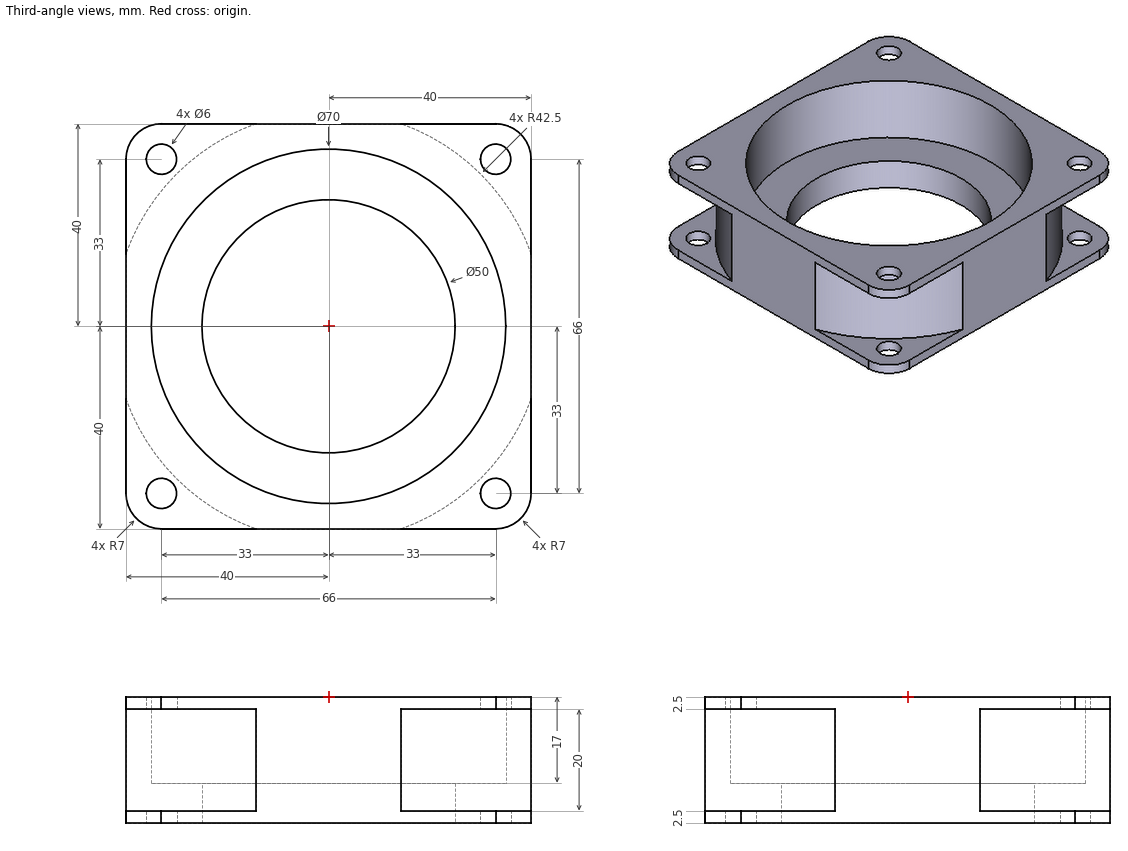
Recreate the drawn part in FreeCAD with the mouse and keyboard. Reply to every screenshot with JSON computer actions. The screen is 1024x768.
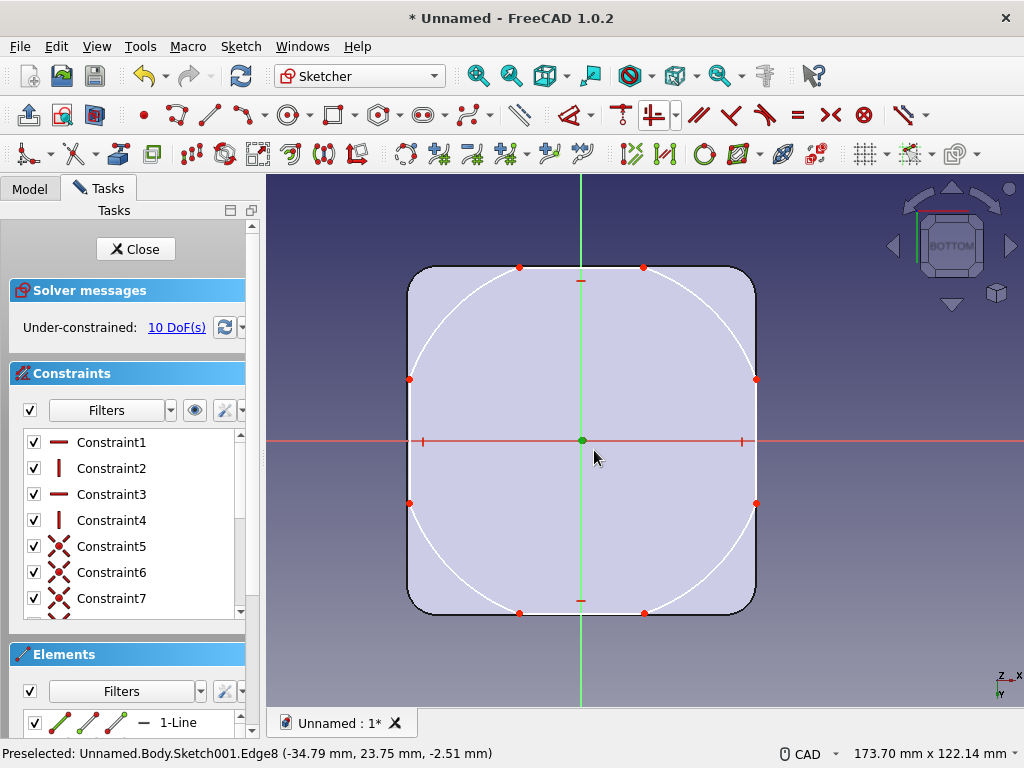
{"action": "left_click", "coordinate": [621, 116]}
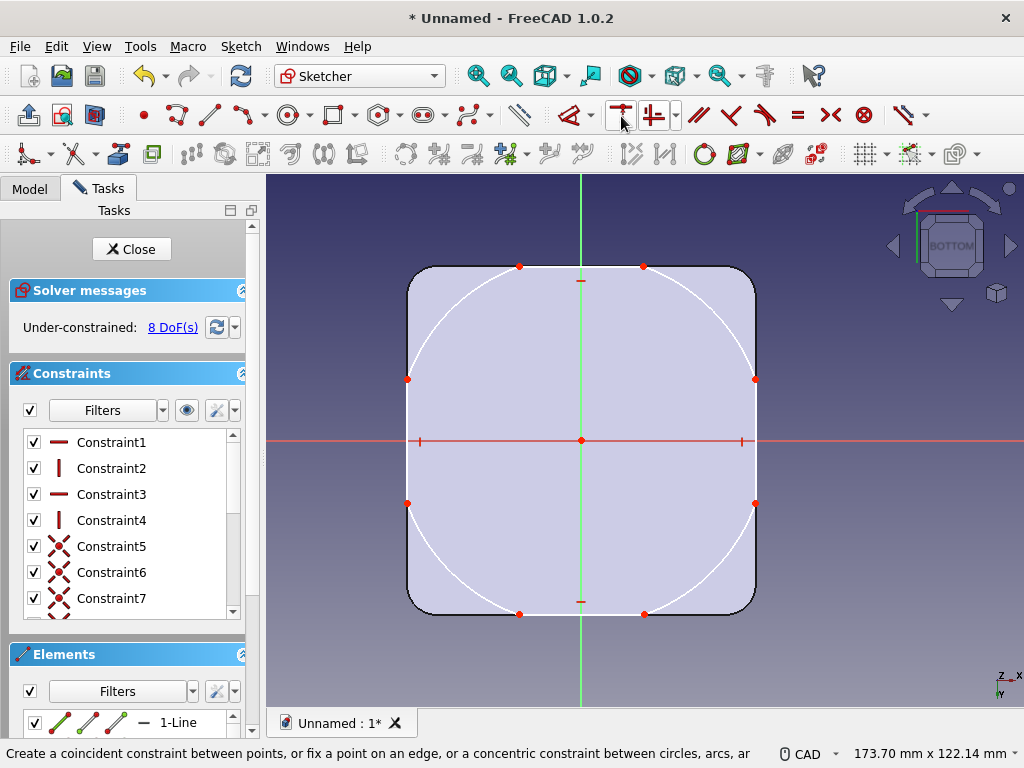
{"action": "left_click", "coordinate": [687, 593]}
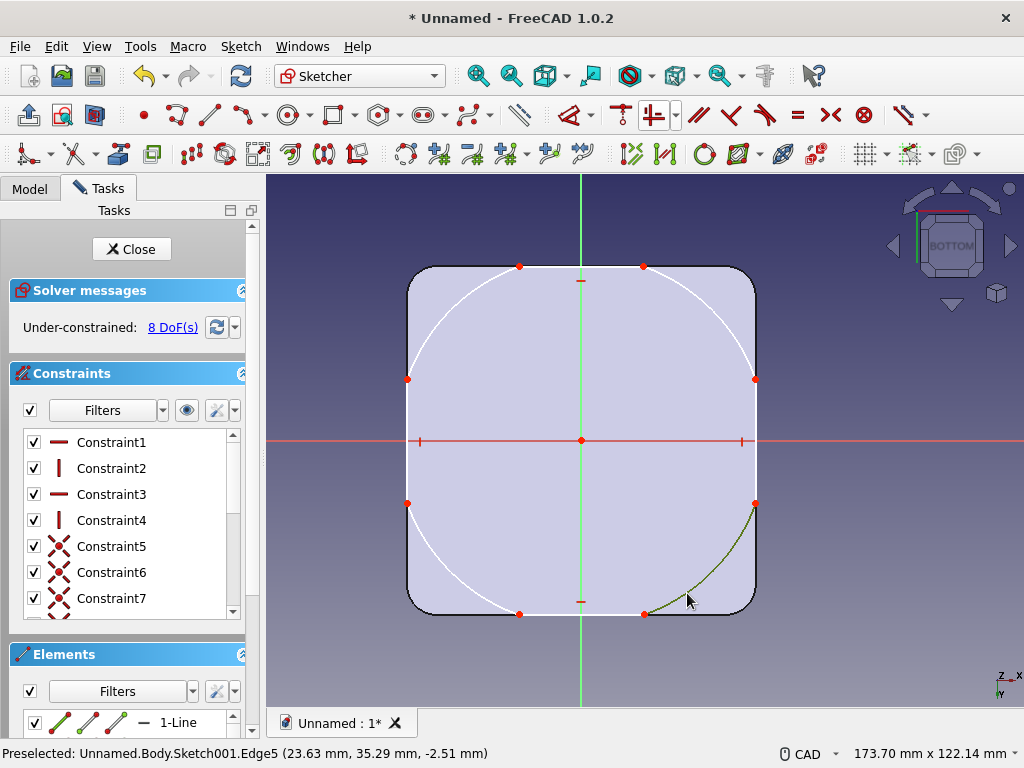
{"action": "left_click", "coordinate": [733, 335]}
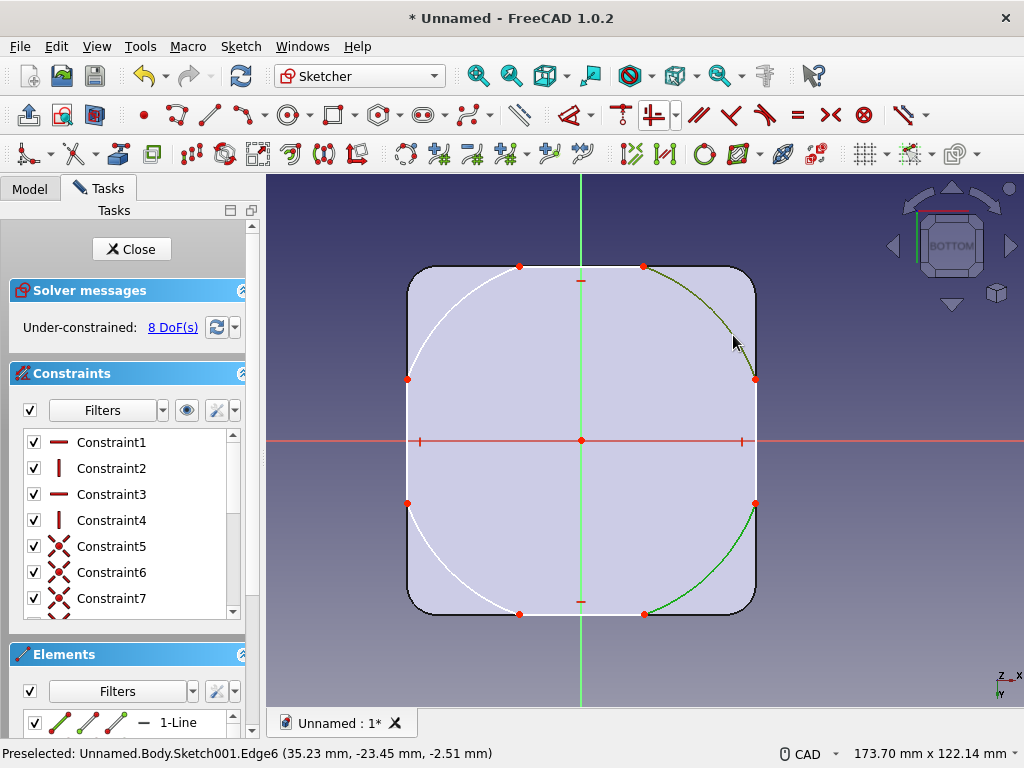
{"action": "left_click", "coordinate": [476, 289]}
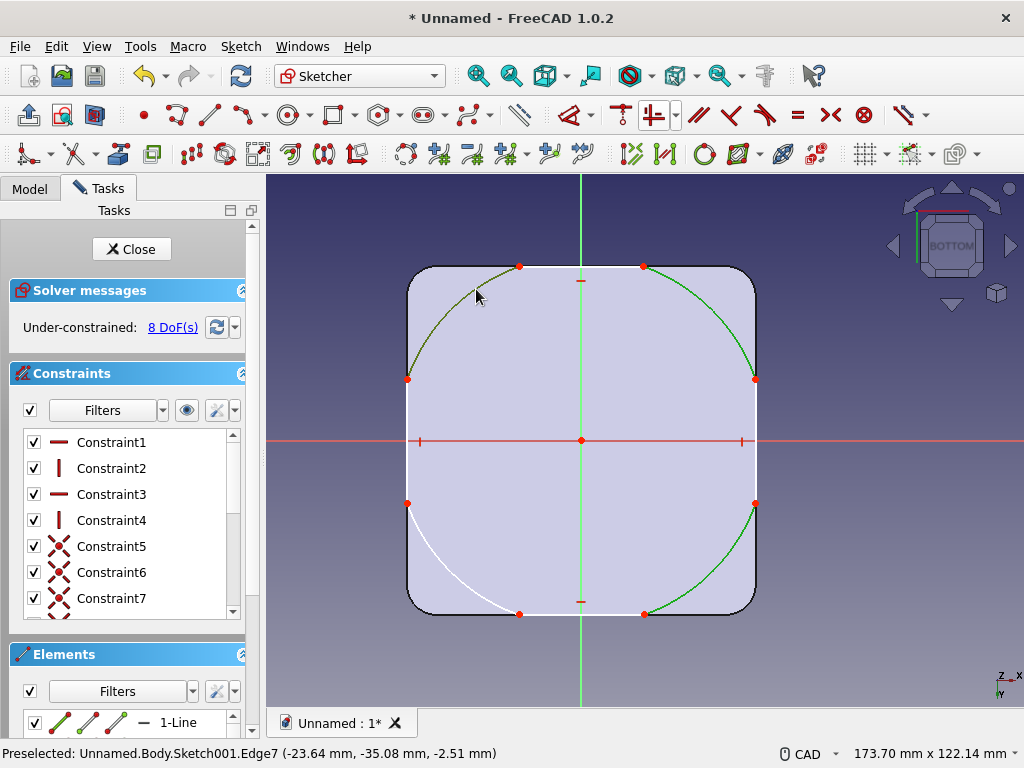
{"action": "left_click", "coordinate": [430, 547]}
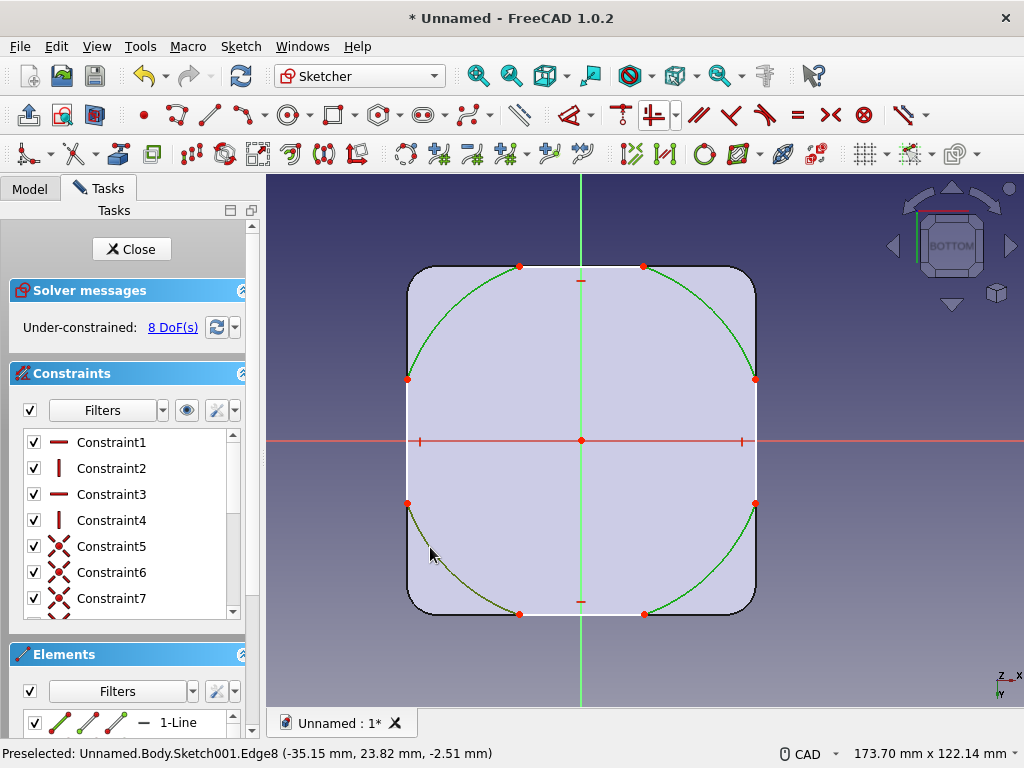
{"action": "left_click", "coordinate": [798, 116]}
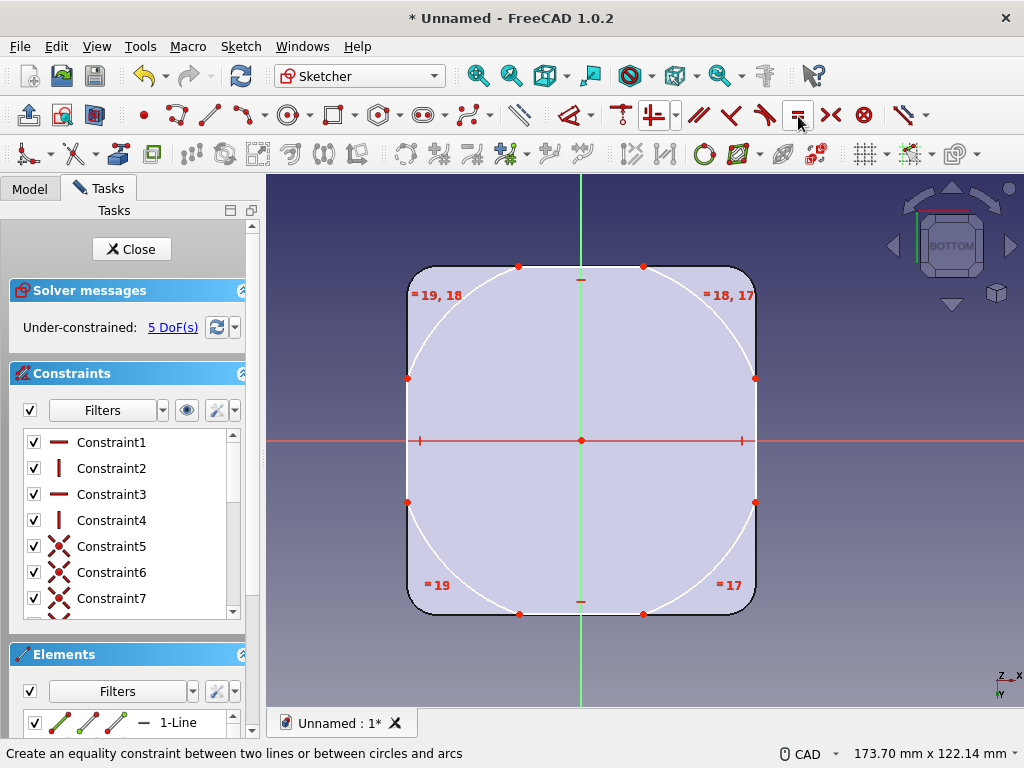
{"action": "left_click", "coordinate": [568, 116]}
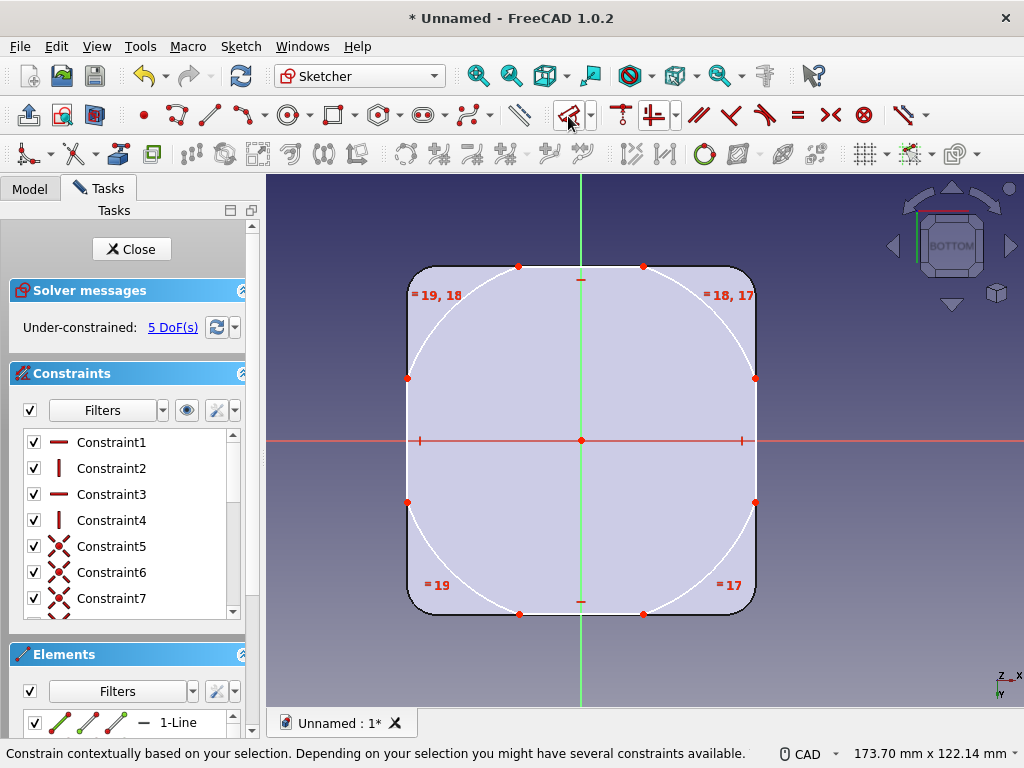
{"action": "left_click", "coordinate": [687, 592]}
{"action": "left_click", "coordinate": [705, 618]}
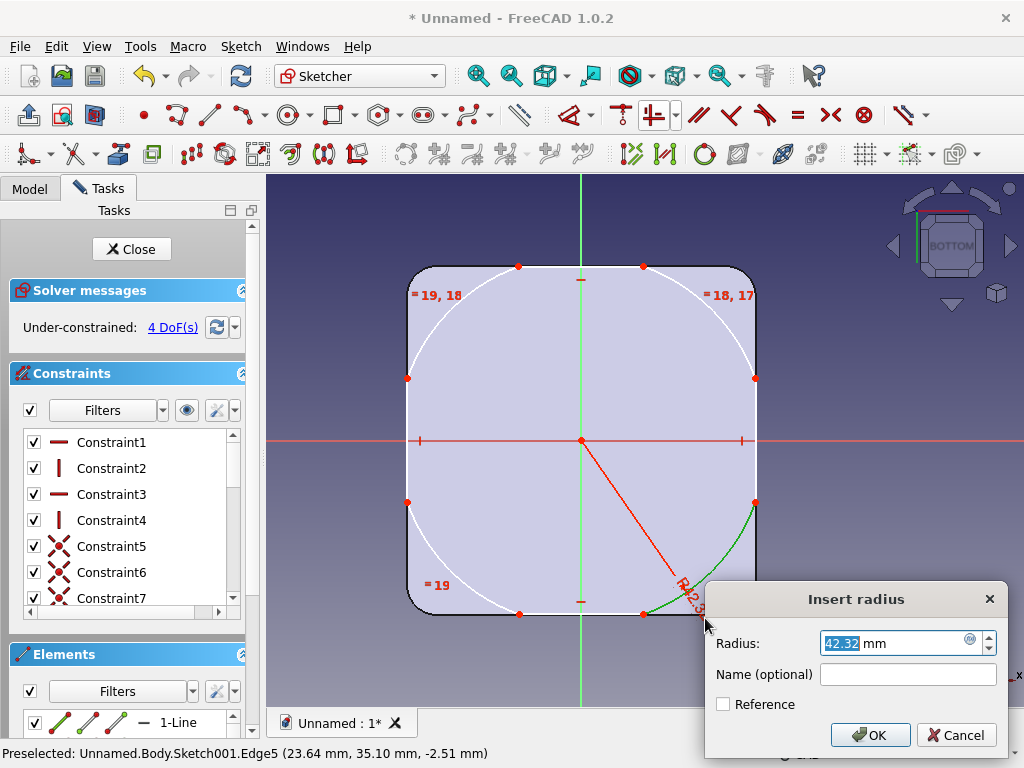
{"action": "type", "text": "42.5"}
{"action": "key", "text": "Return"}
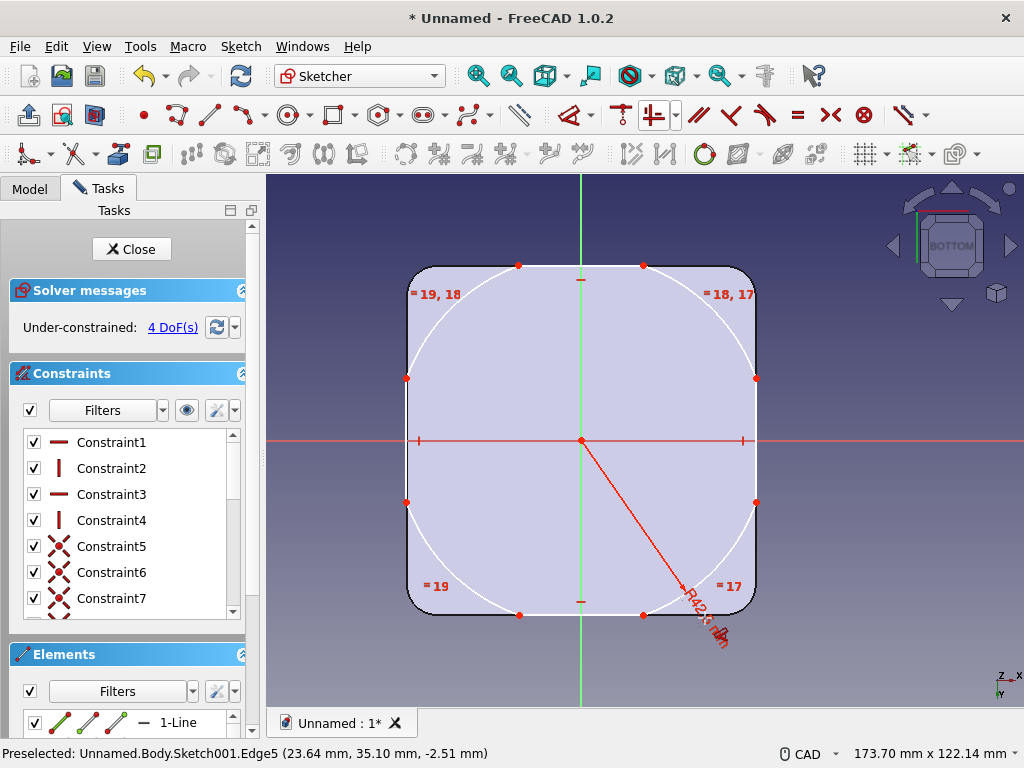
{"action": "left_click", "coordinate": [519, 615]}
{"action": "left_click", "coordinate": [485, 528]}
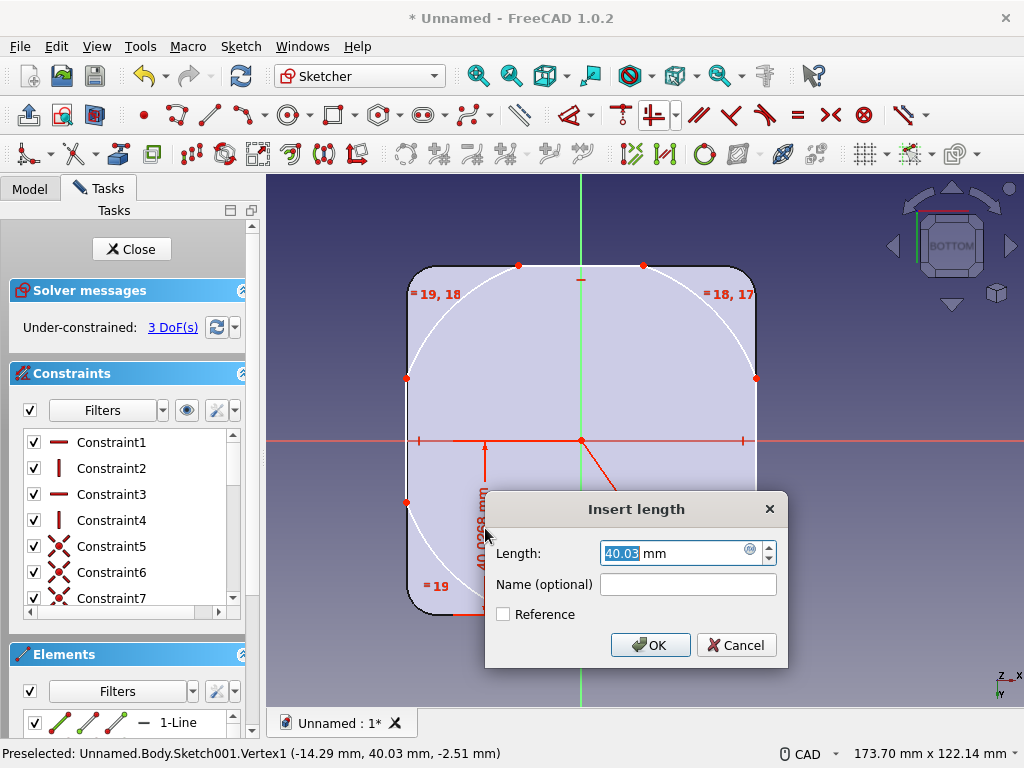
{"action": "type", "text": "40"}
{"action": "key", "text": "Return"}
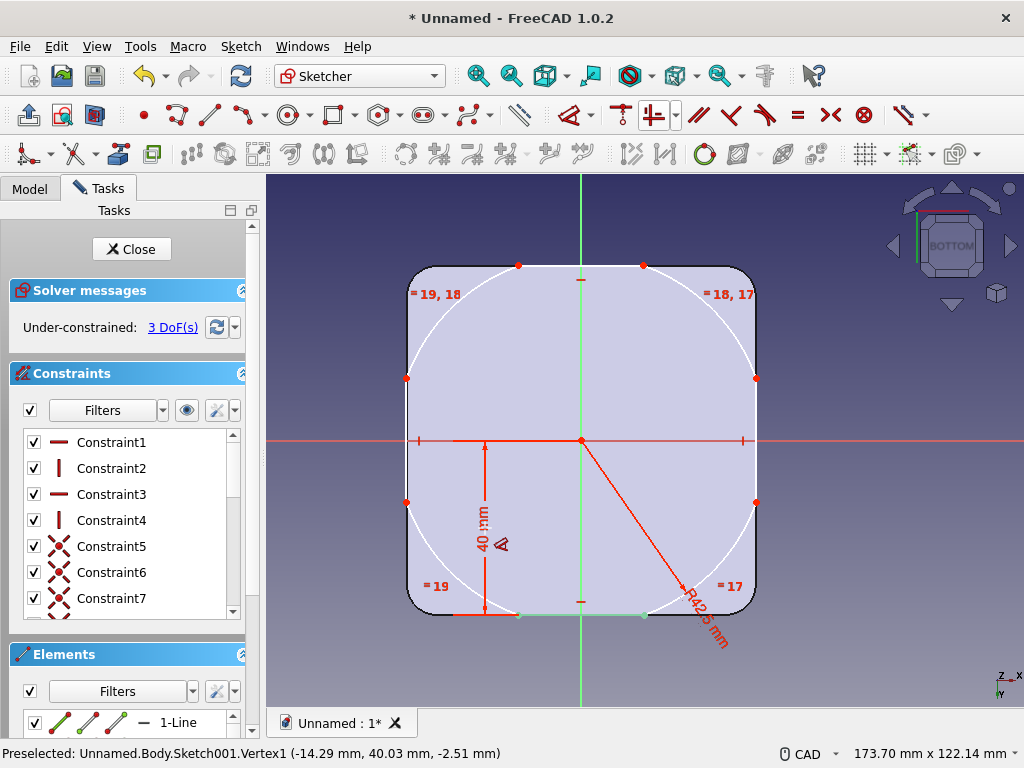
{"action": "left_click", "coordinate": [756, 502]}
{"action": "left_click", "coordinate": [669, 536]}